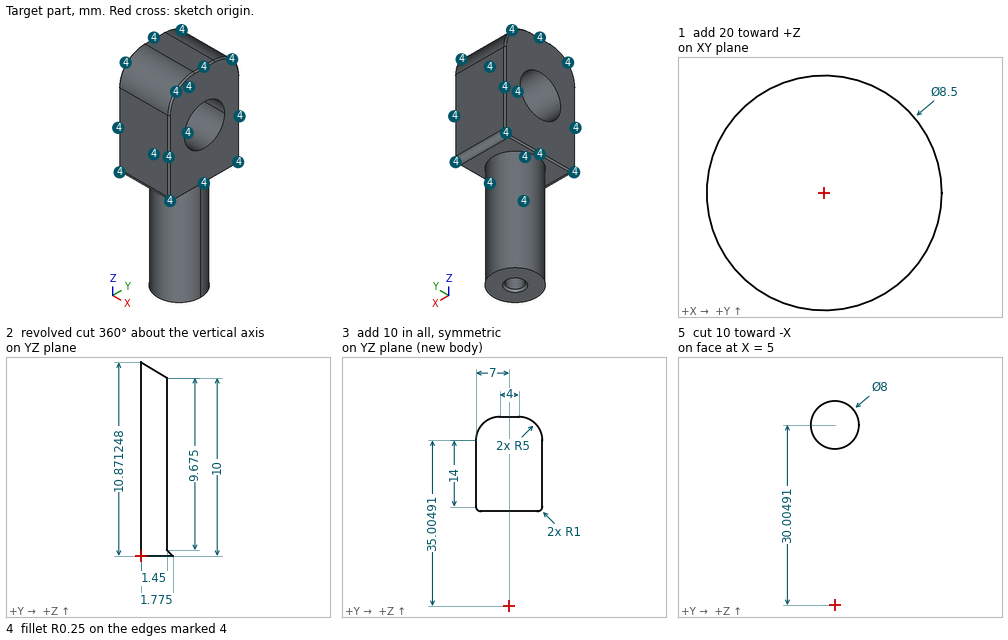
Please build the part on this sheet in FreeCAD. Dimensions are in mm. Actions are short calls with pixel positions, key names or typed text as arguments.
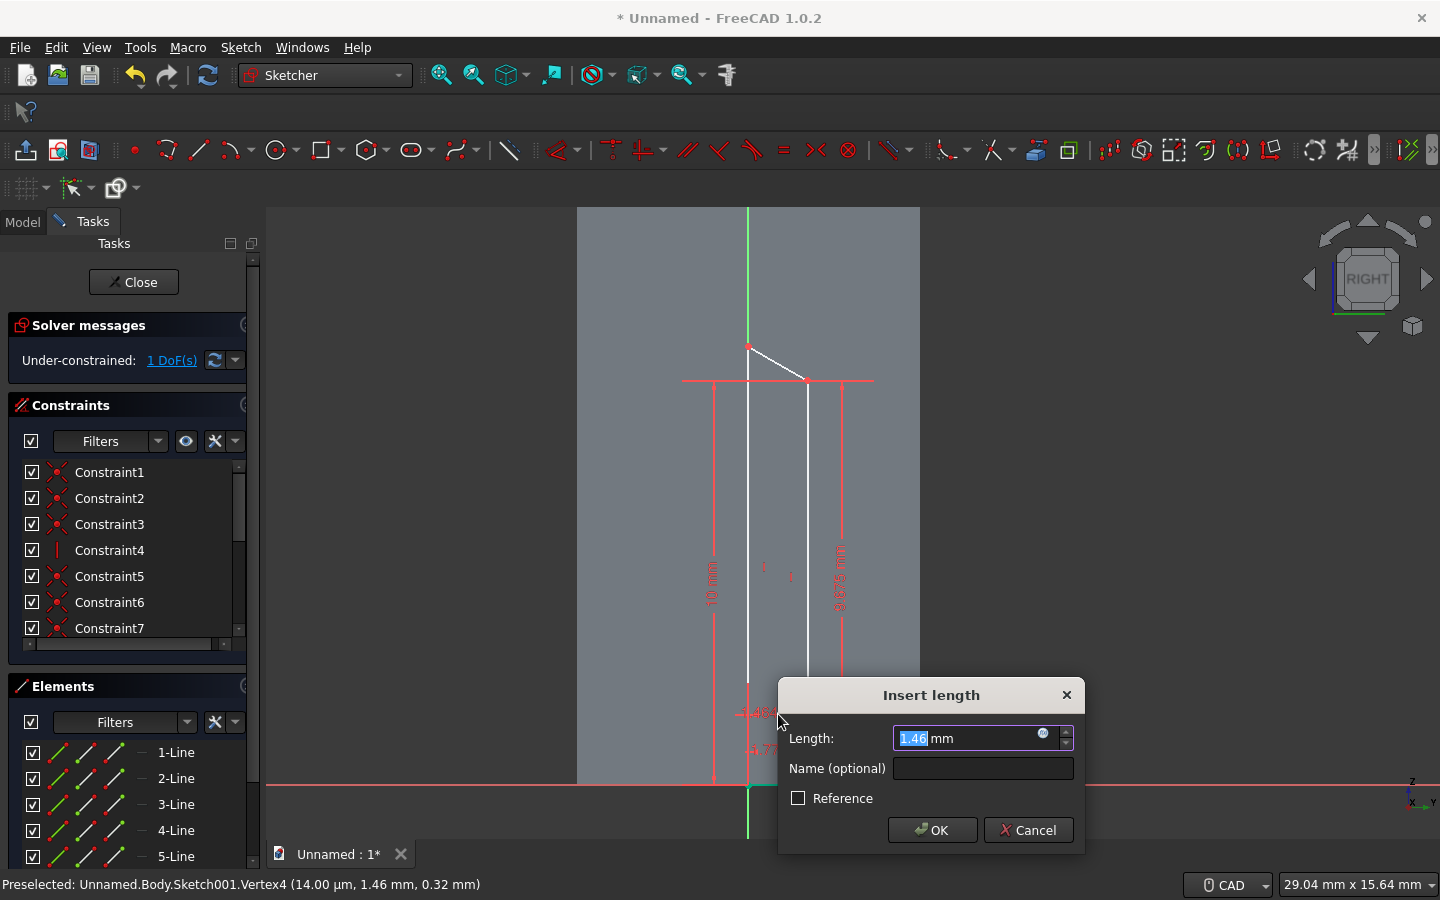
text(1.45)
key(Return)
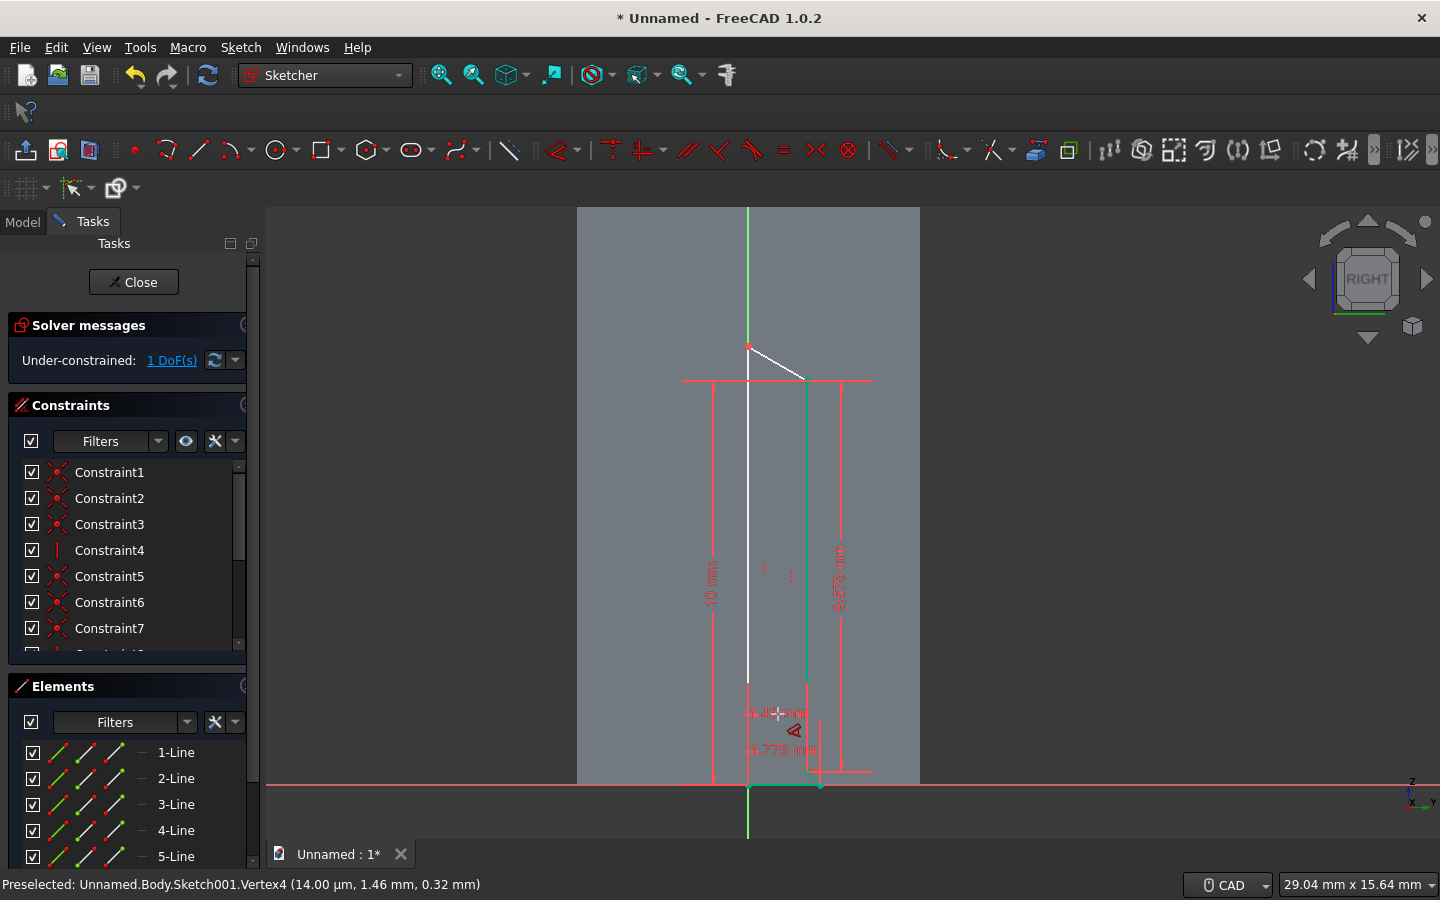
click(748, 478)
click(714, 465)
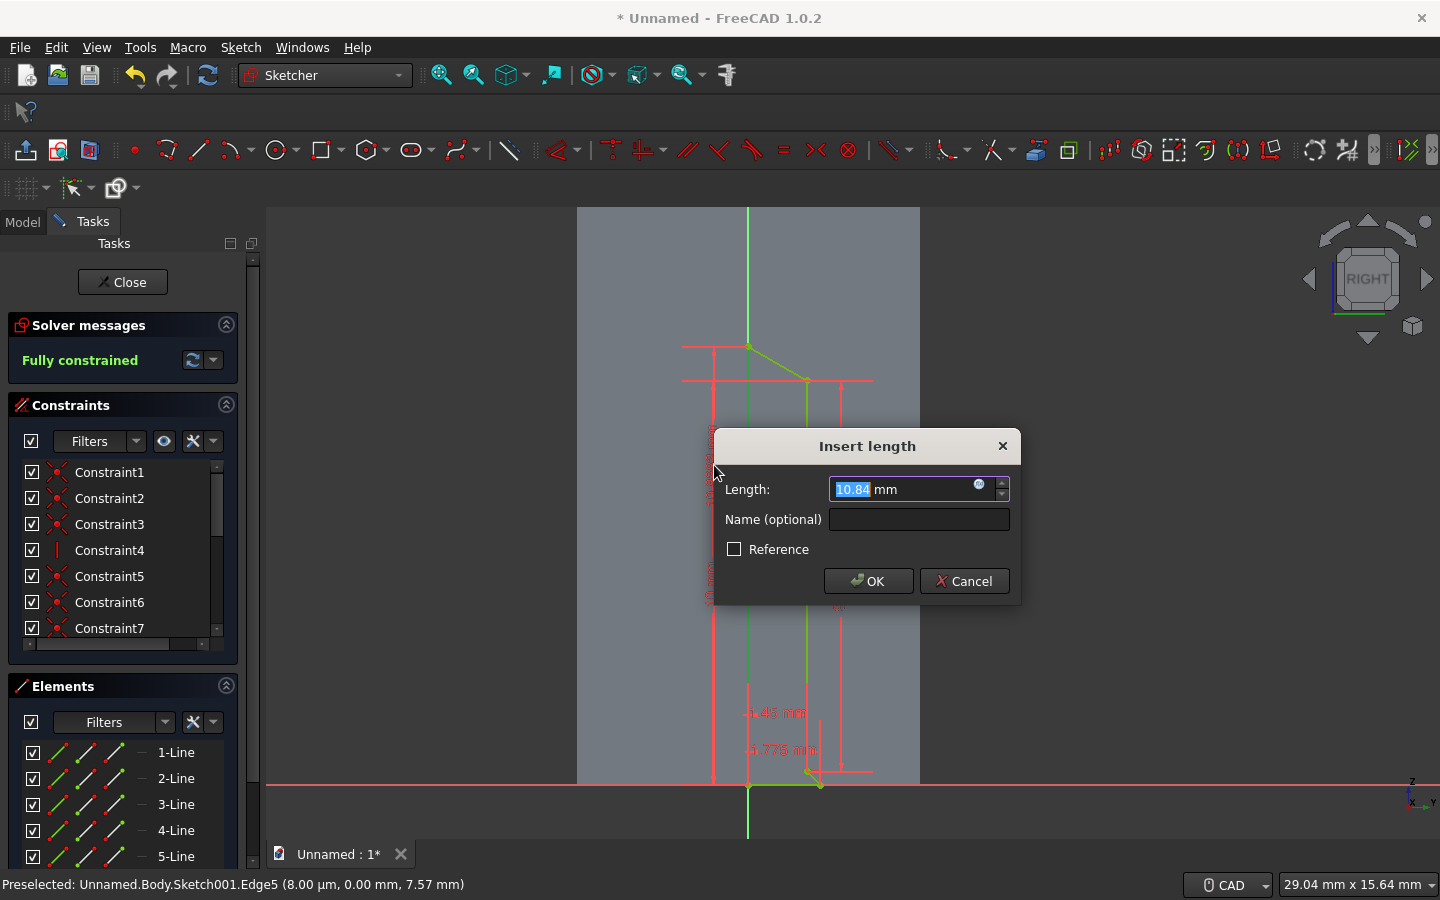
text(10.871248)
key(Return)
key(Escape)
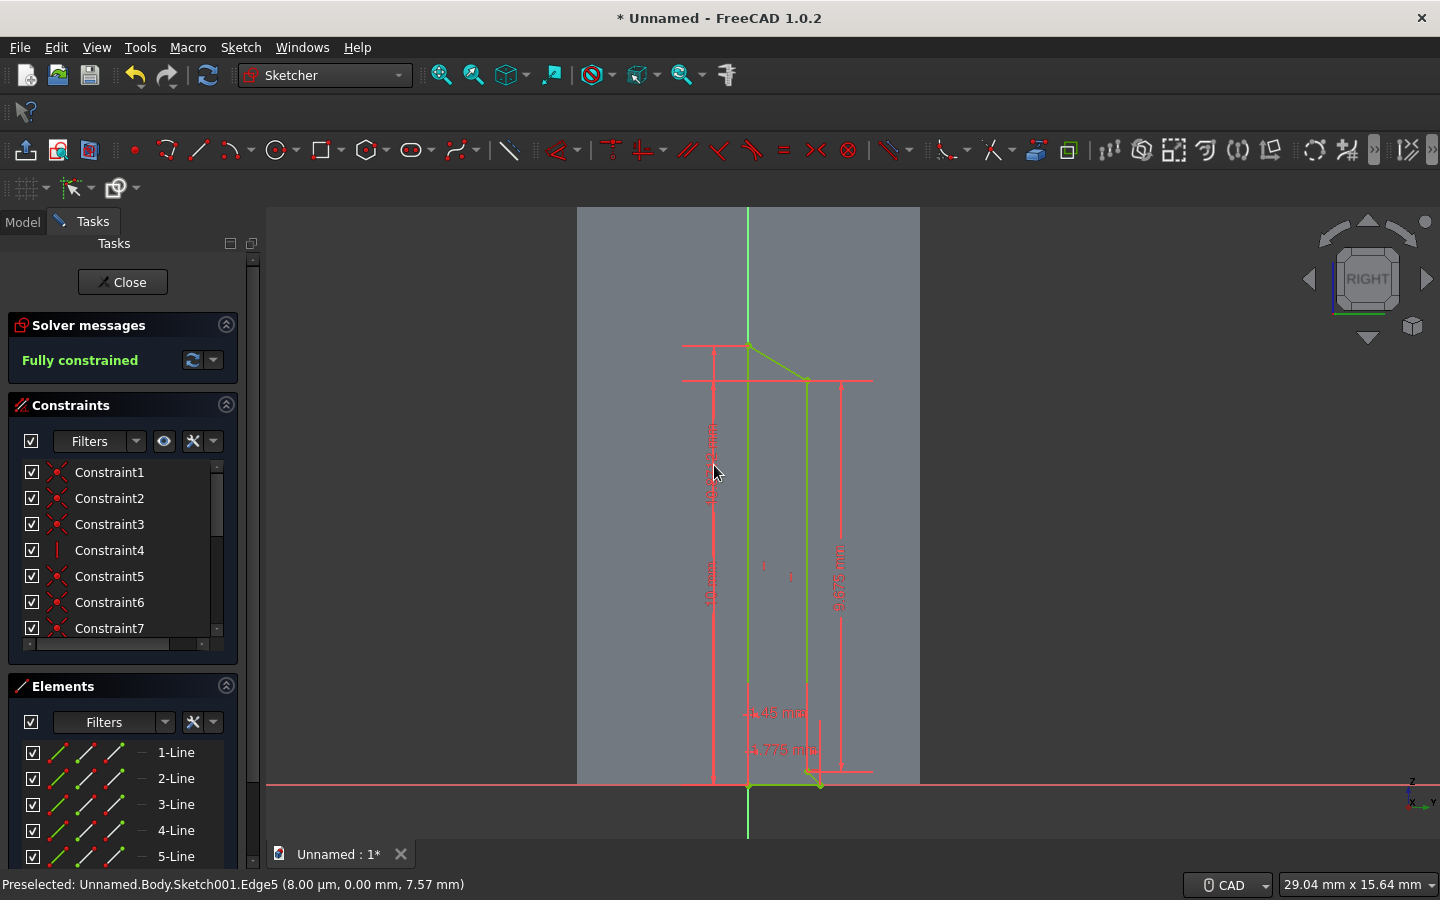
click(123, 282)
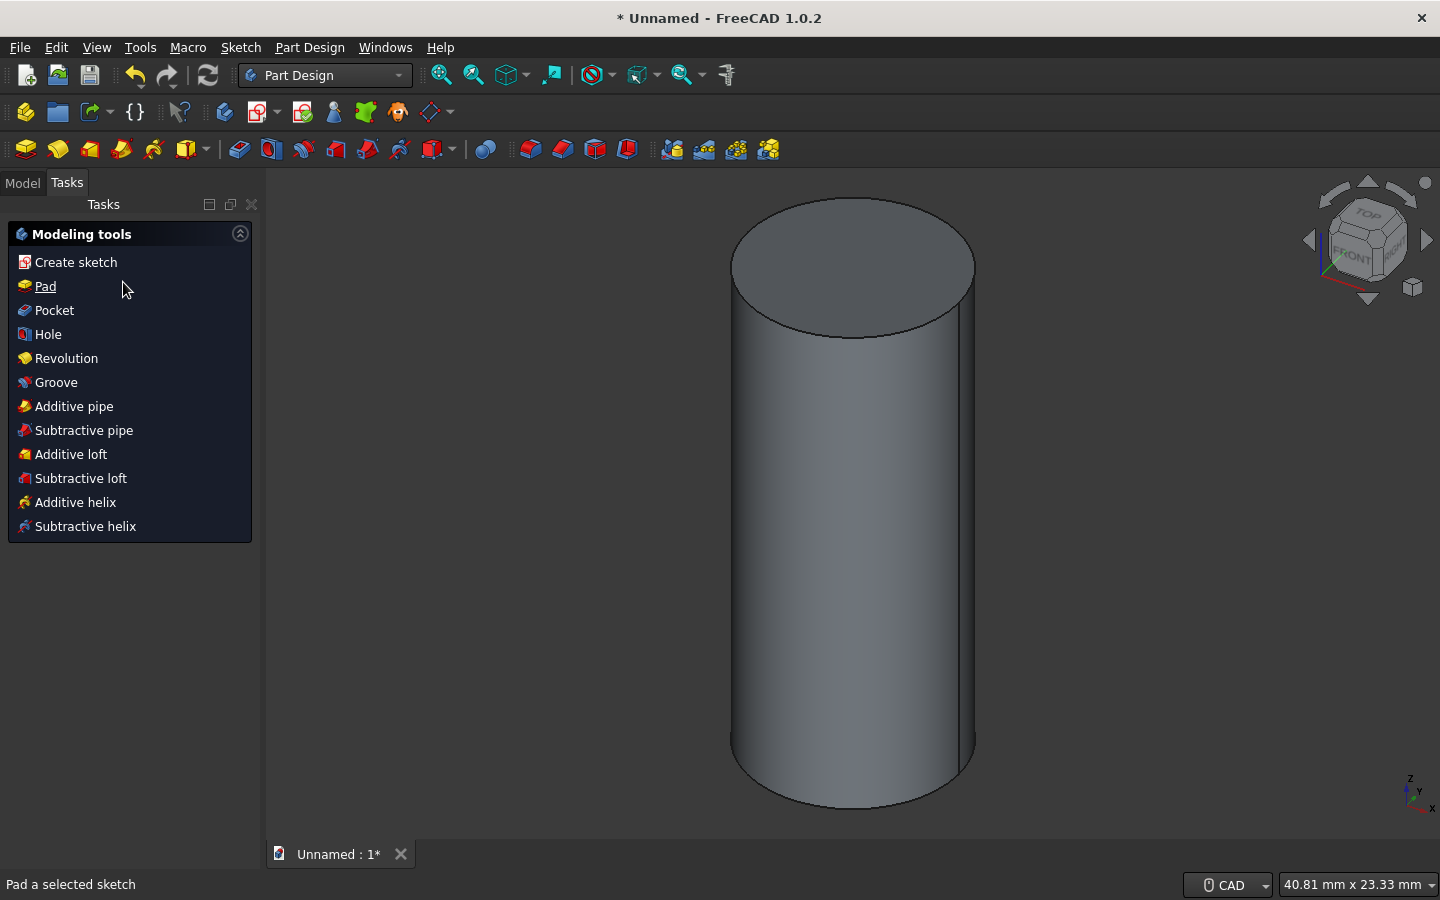
click(304, 150)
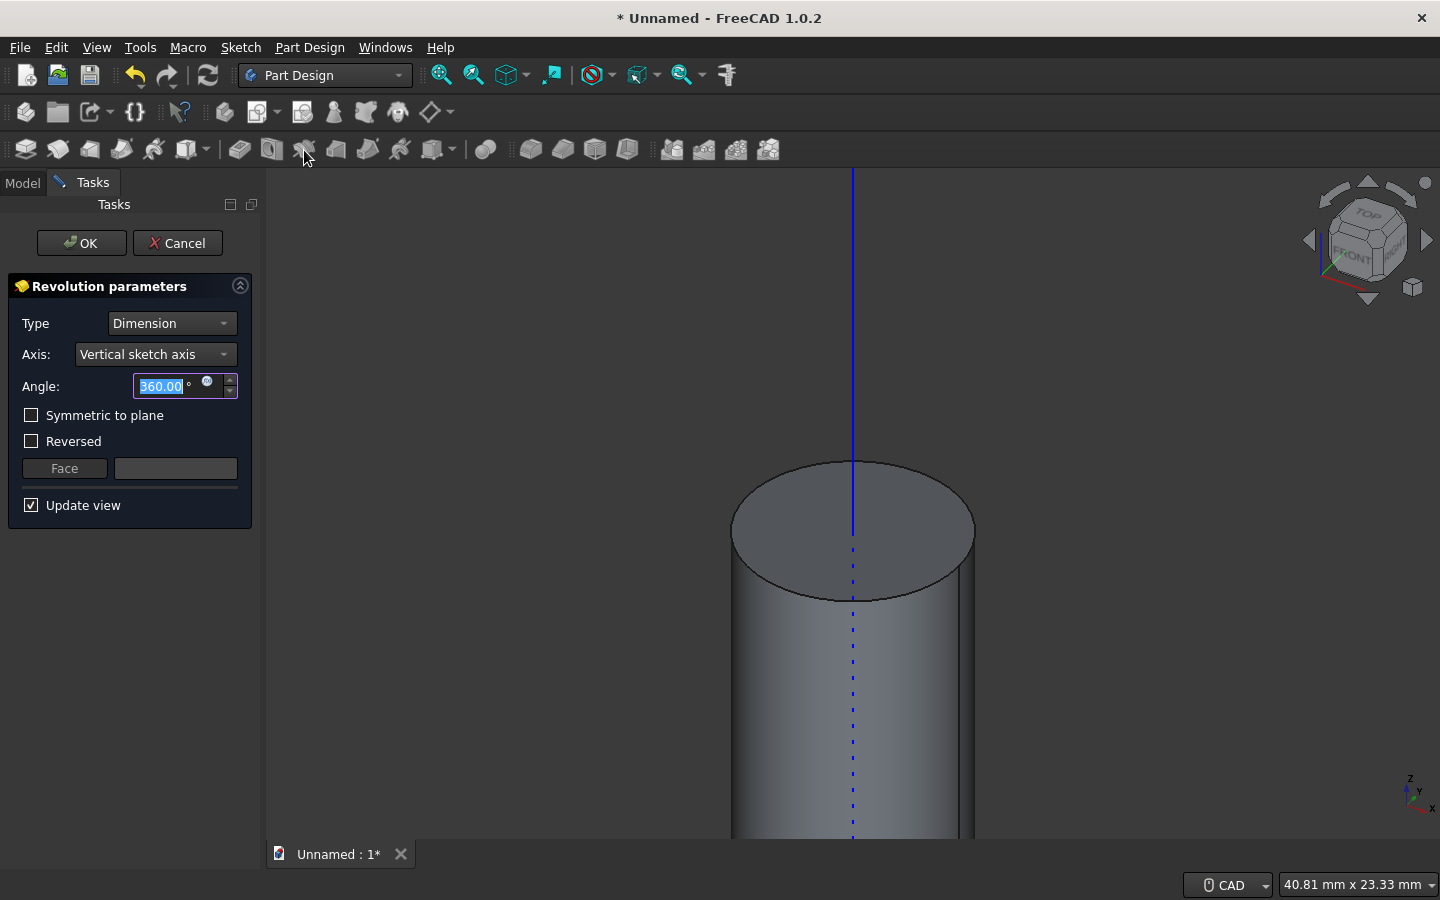
click(82, 243)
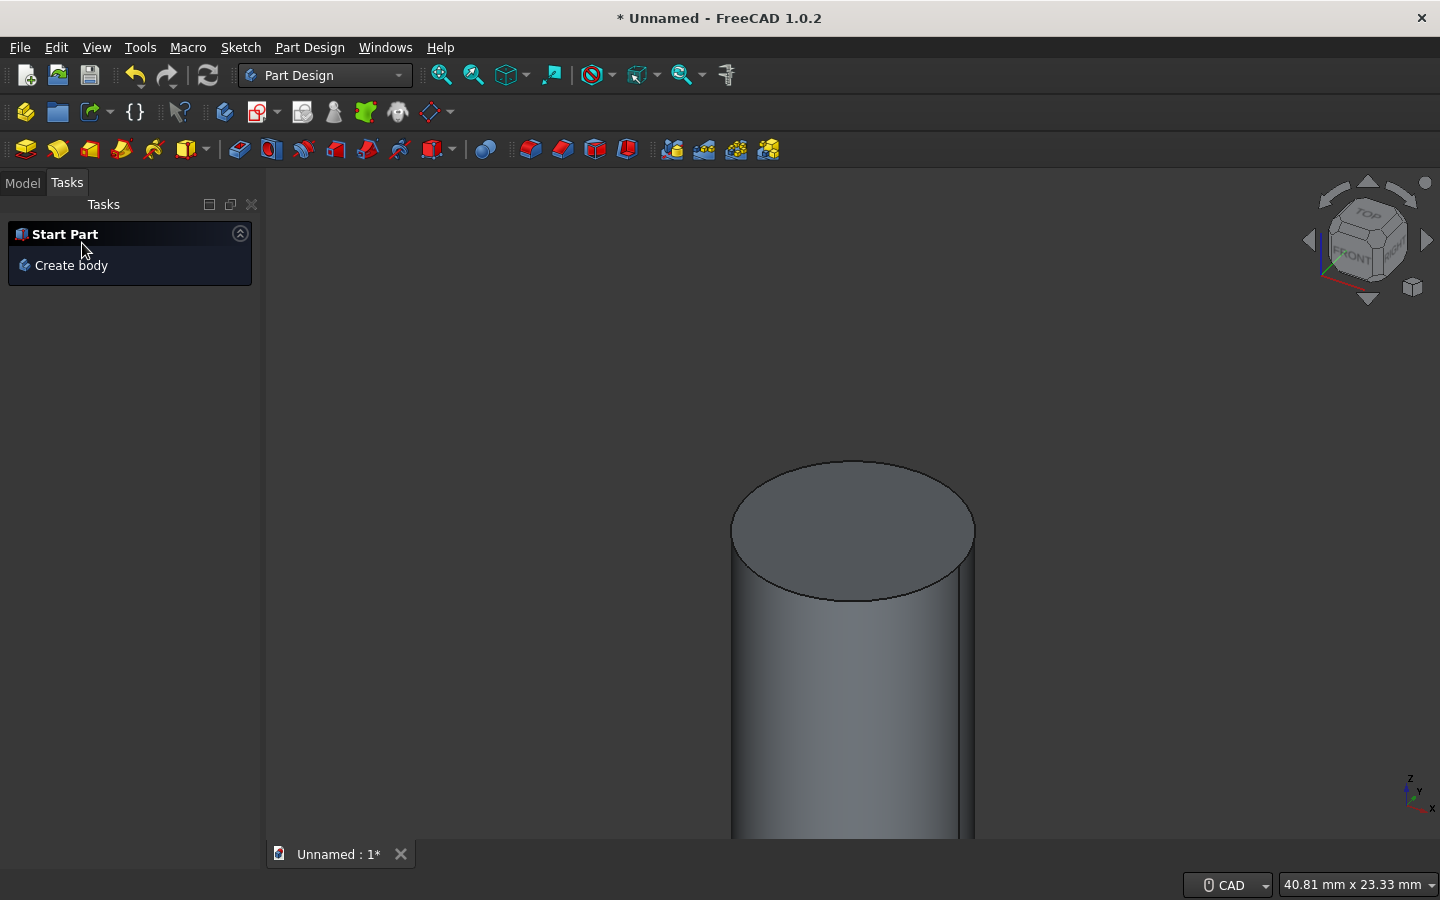
key(v)
key(f)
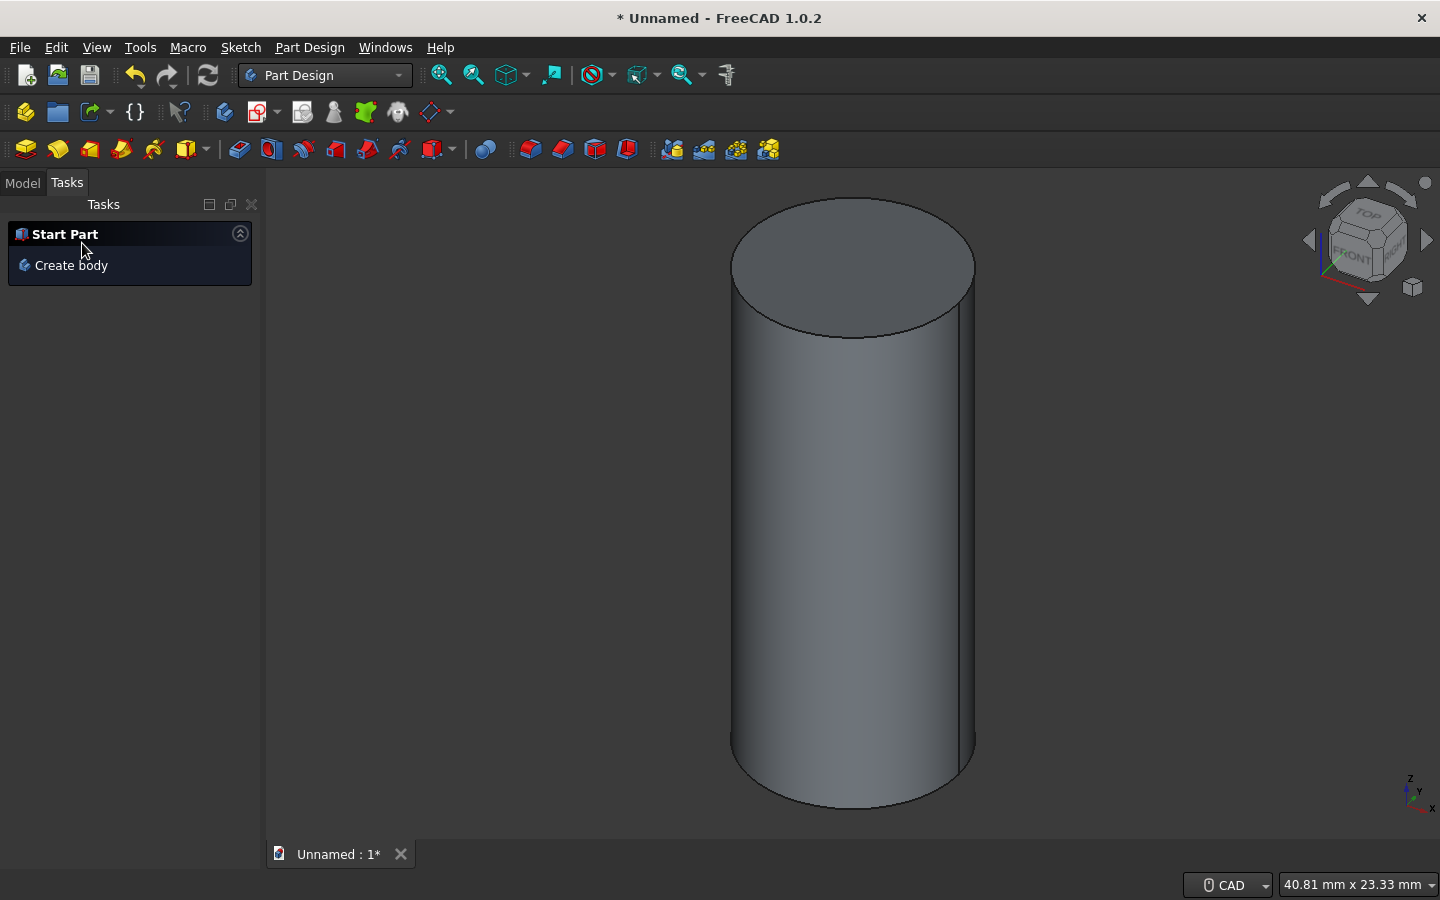
click(226, 112)